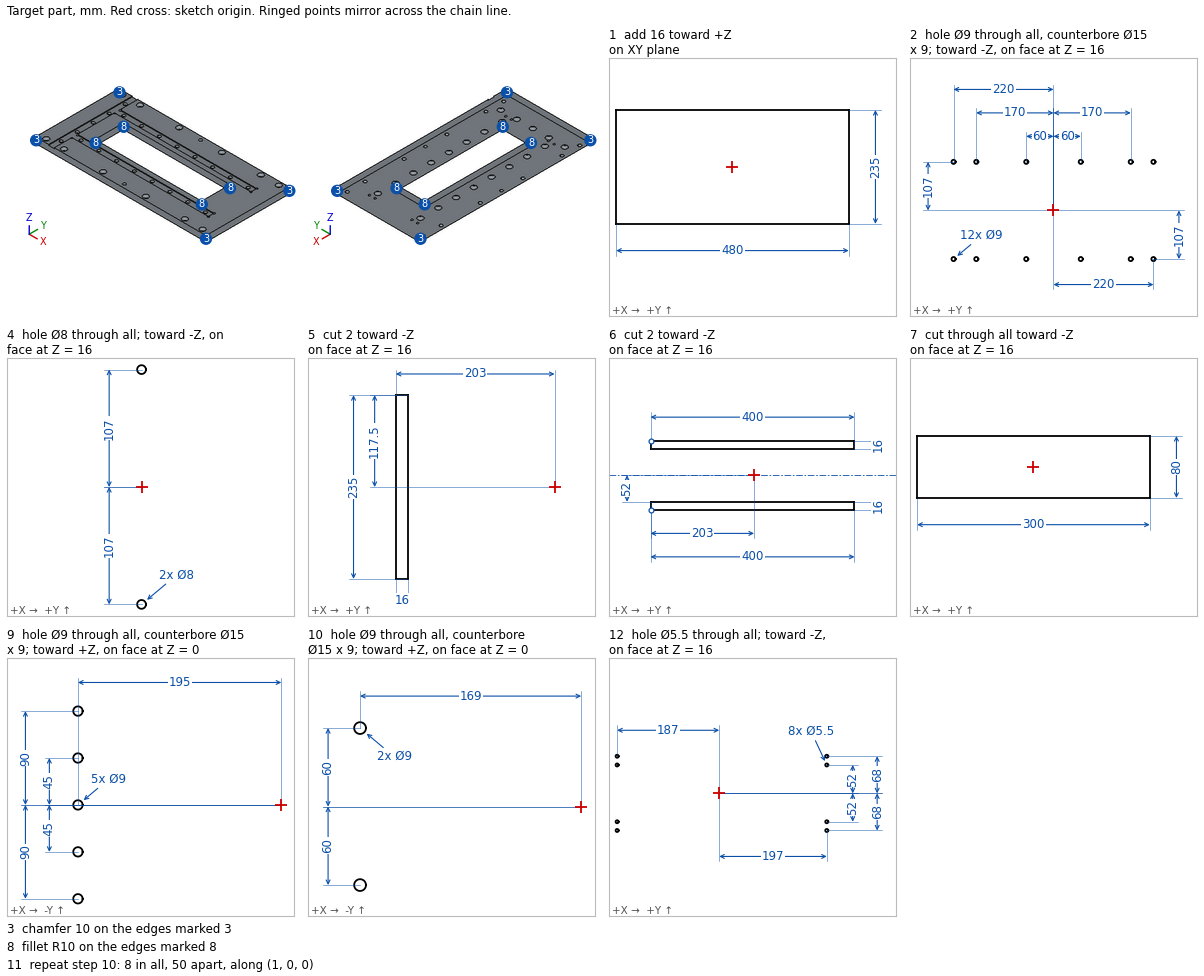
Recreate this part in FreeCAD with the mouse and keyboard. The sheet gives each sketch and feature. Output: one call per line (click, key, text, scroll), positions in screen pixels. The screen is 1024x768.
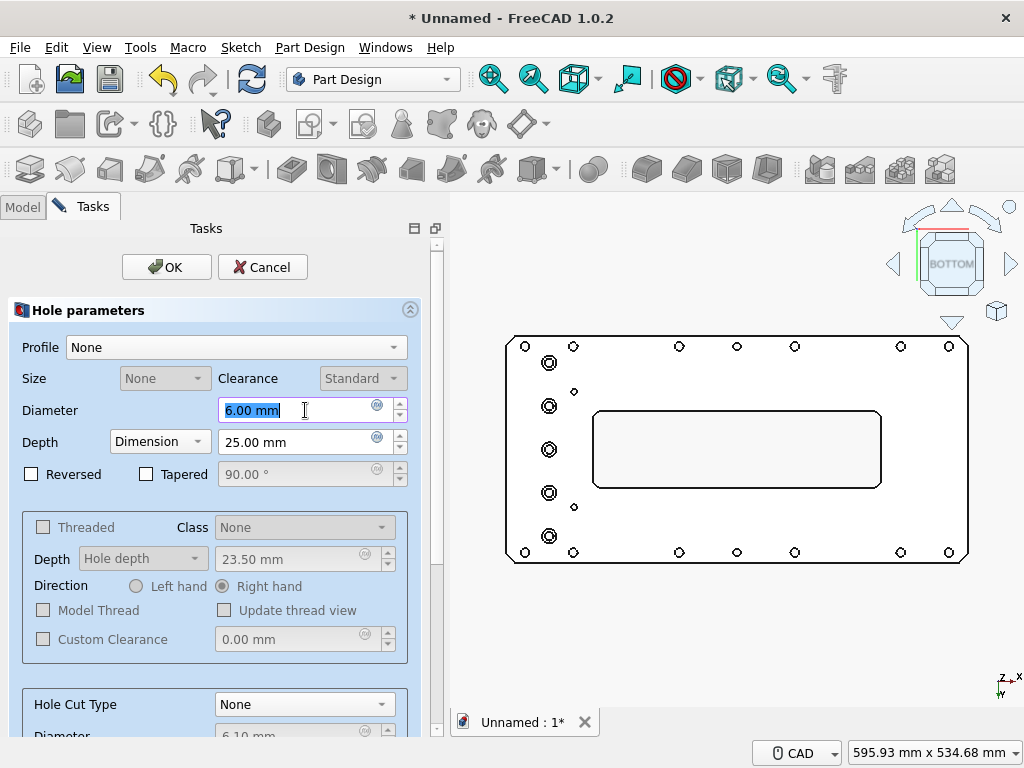
text(9)
key(Tab)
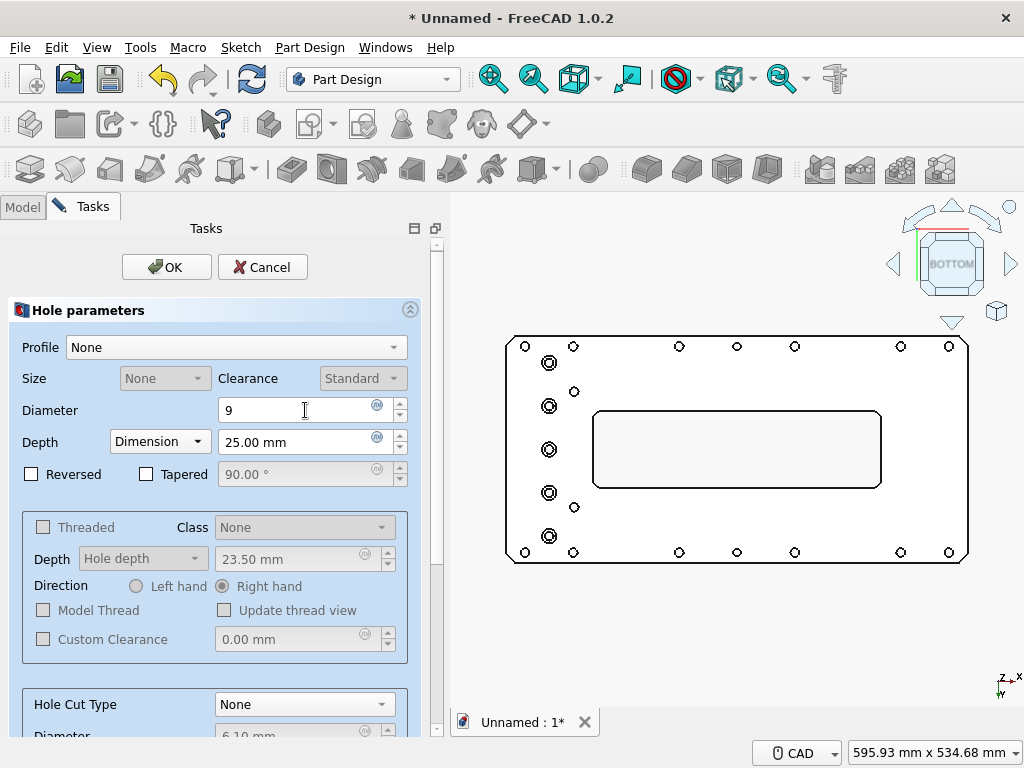
click(161, 442)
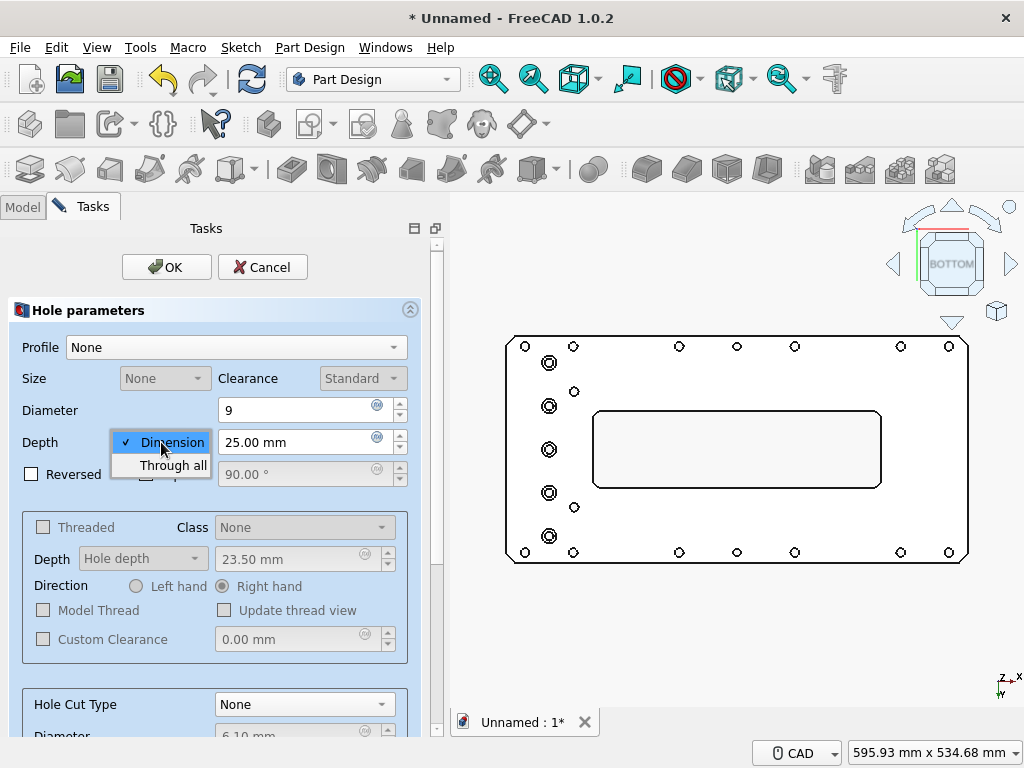
click(160, 466)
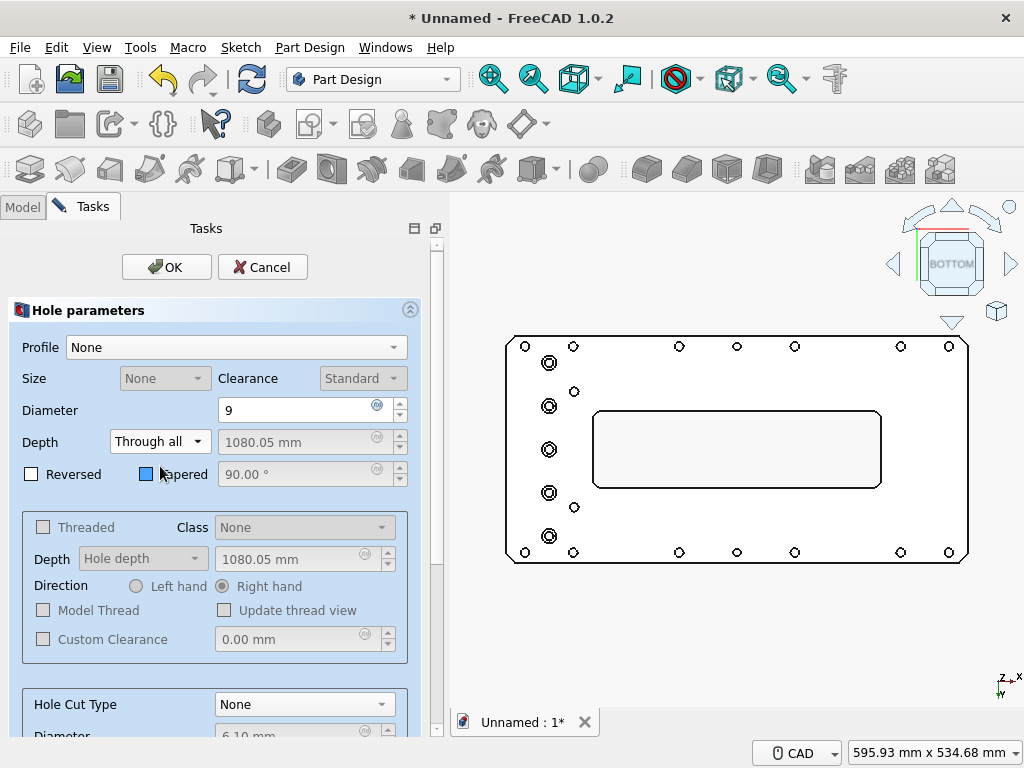
click(306, 704)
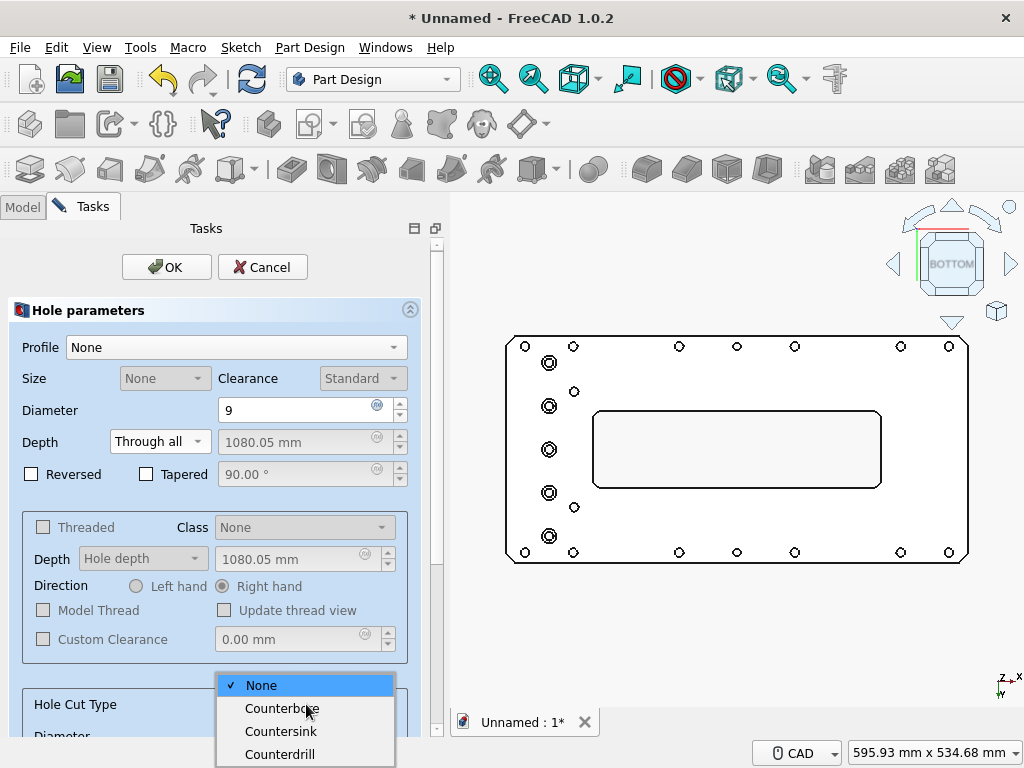
click(304, 708)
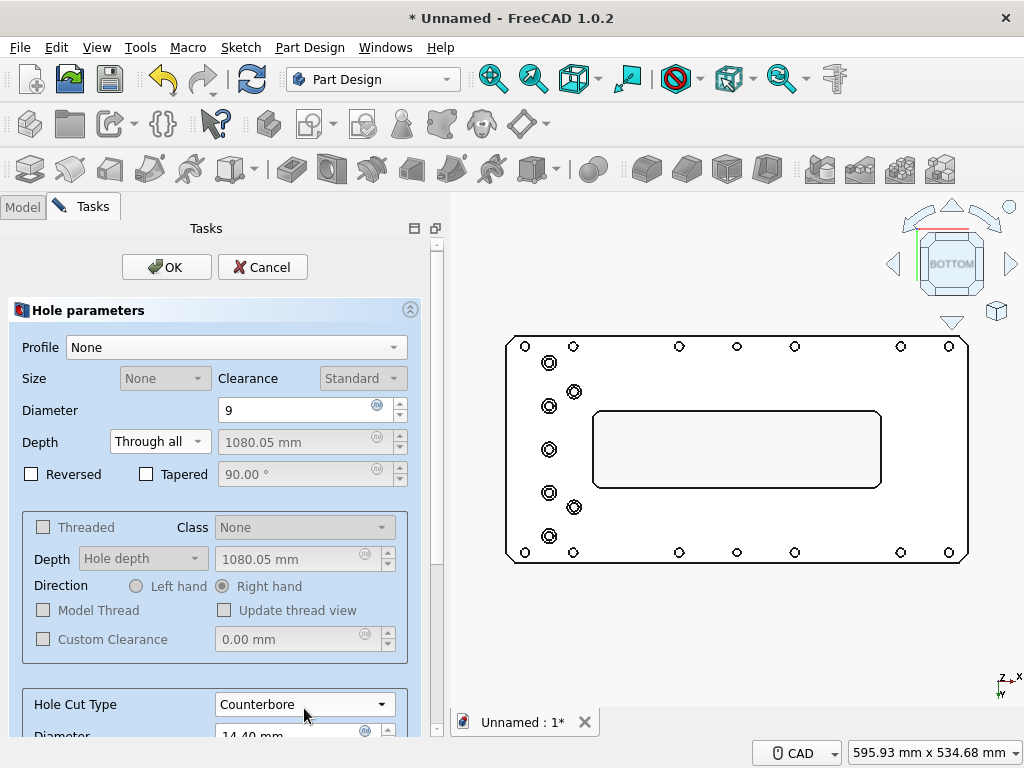
scroll(437, 487, down, 2)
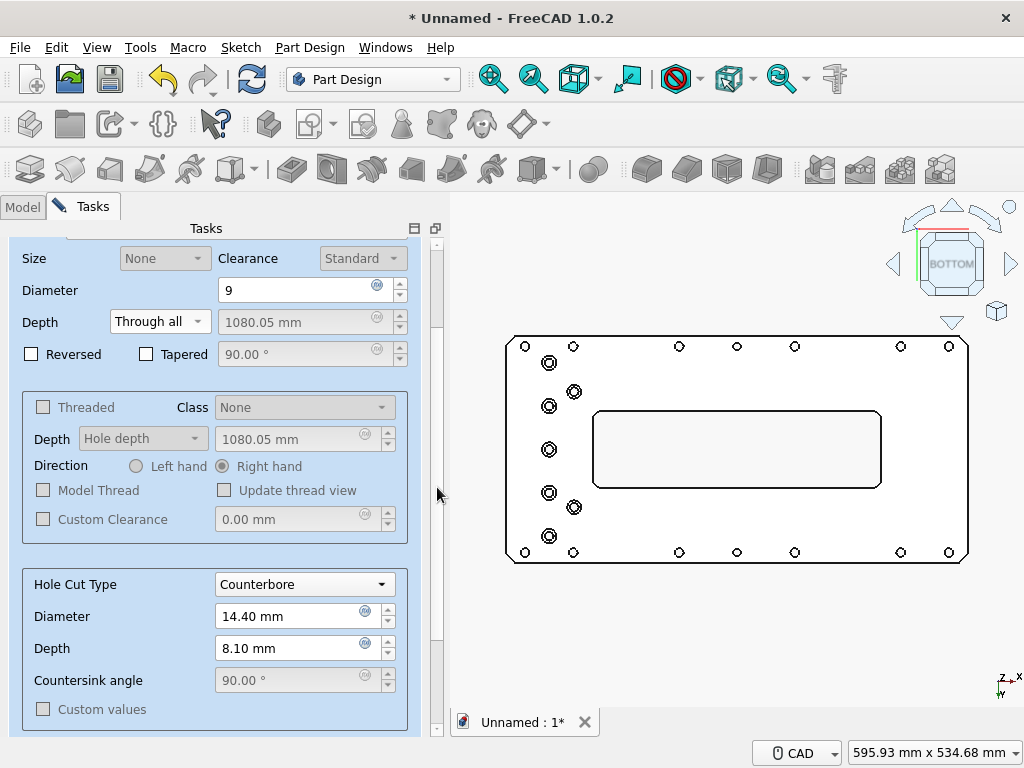
triple_click(298, 616)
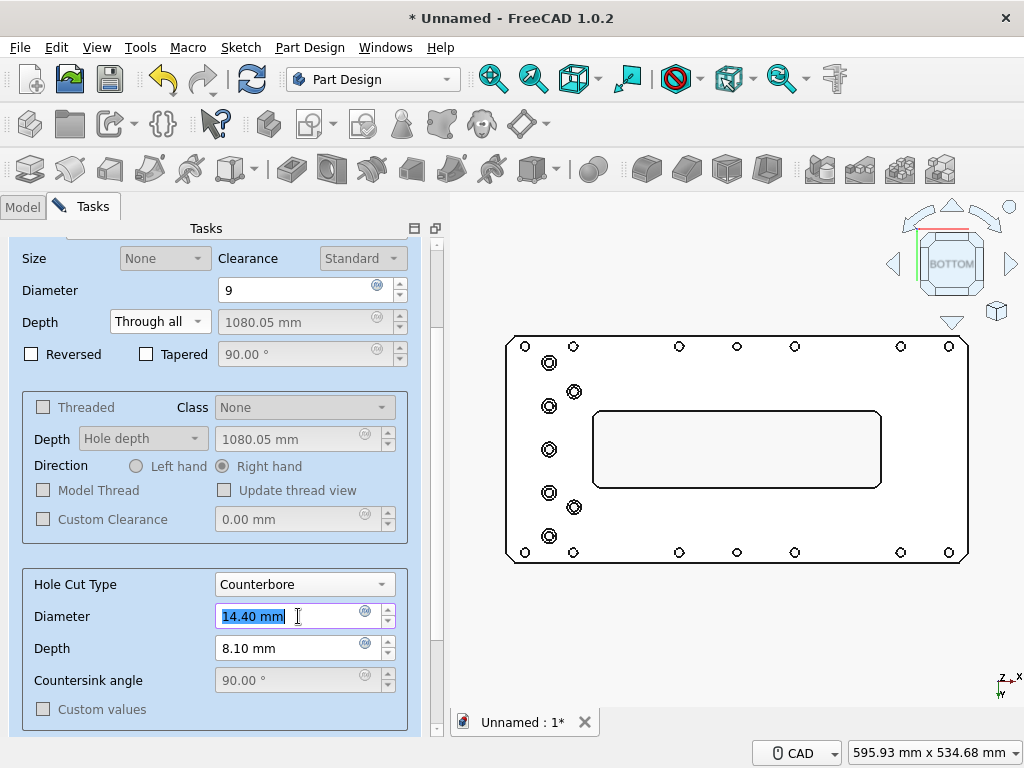
text(15)
key(Tab)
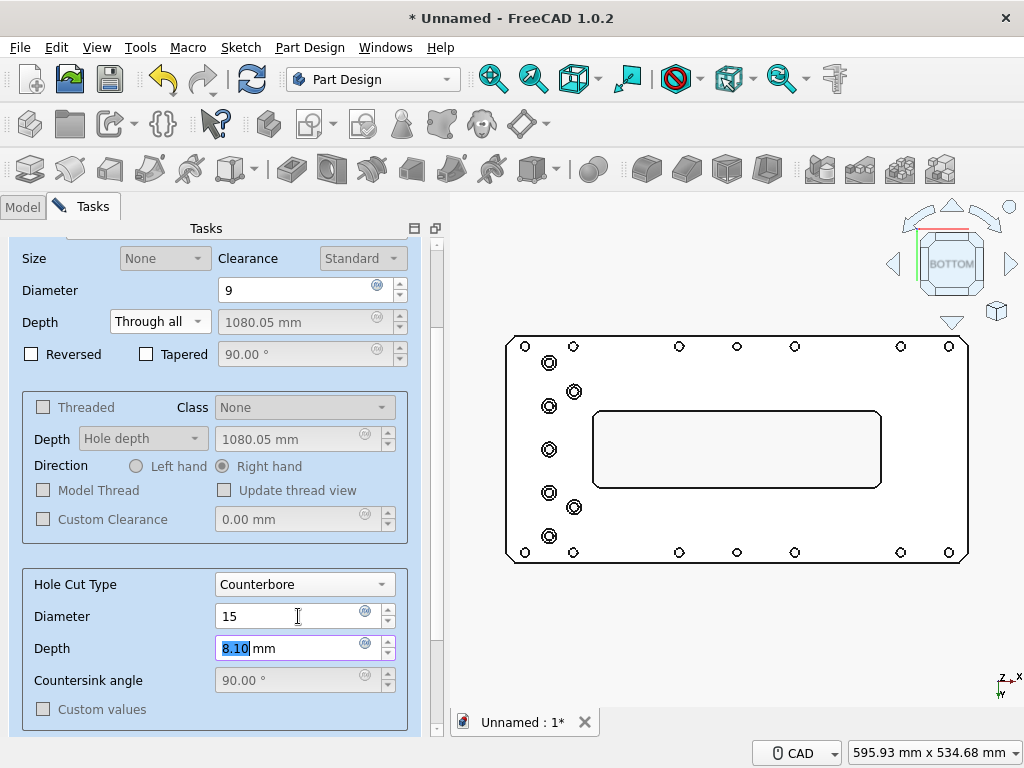
text(9)
key(Tab)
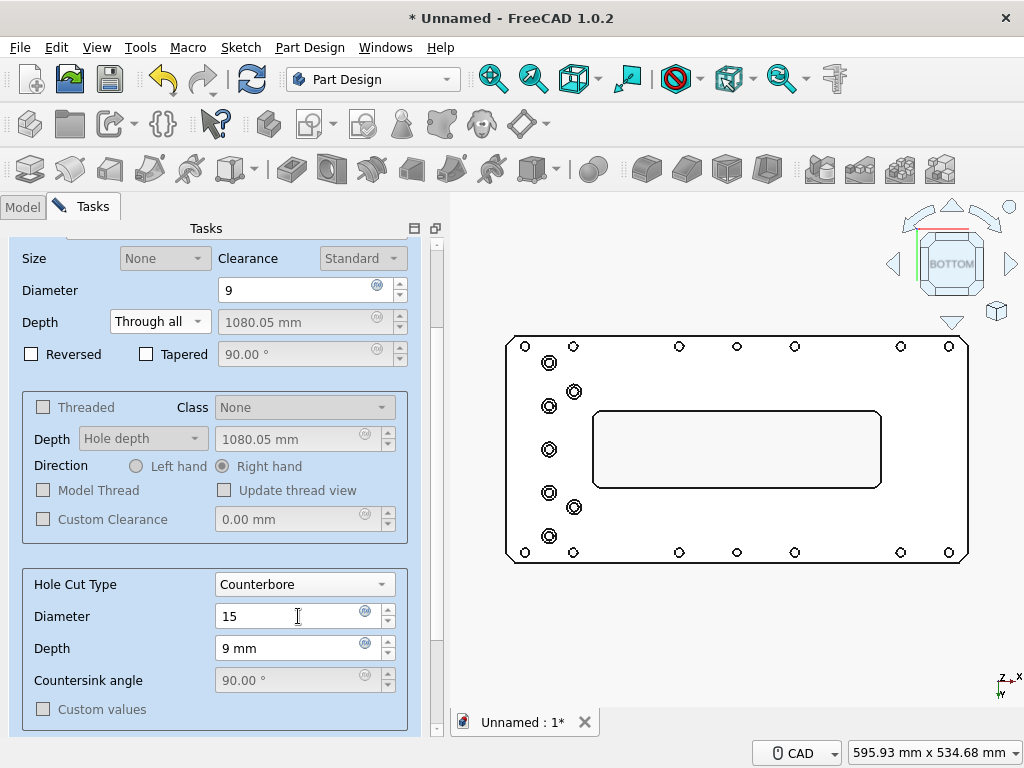
scroll(437, 487, up, 3)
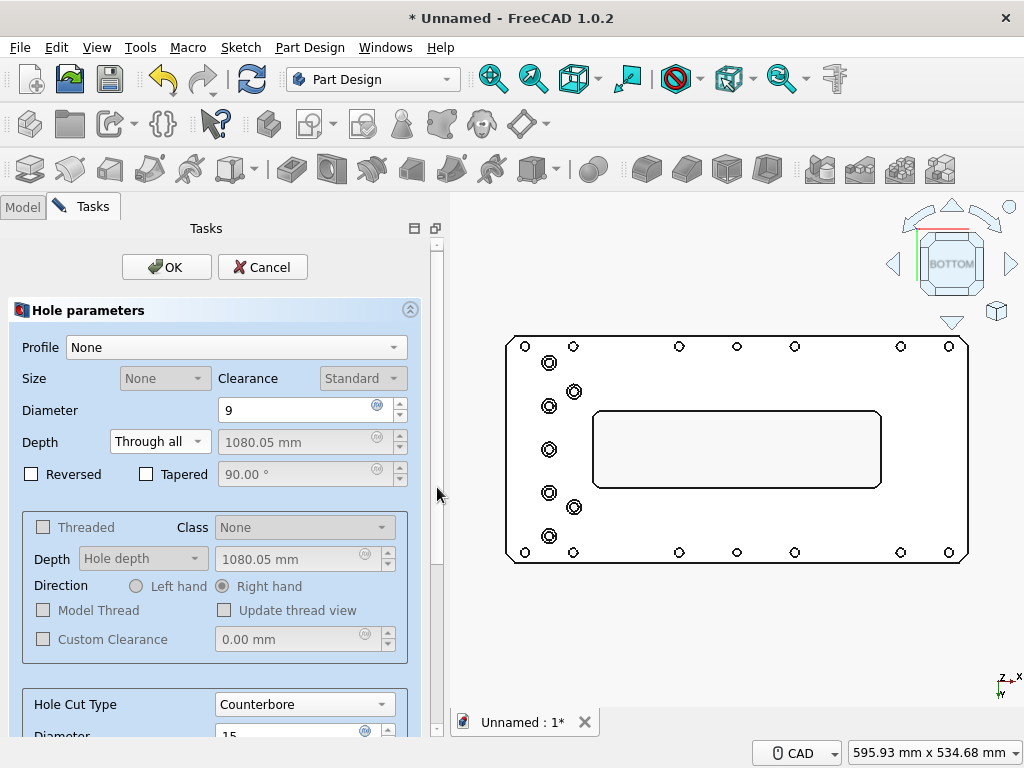
click(167, 267)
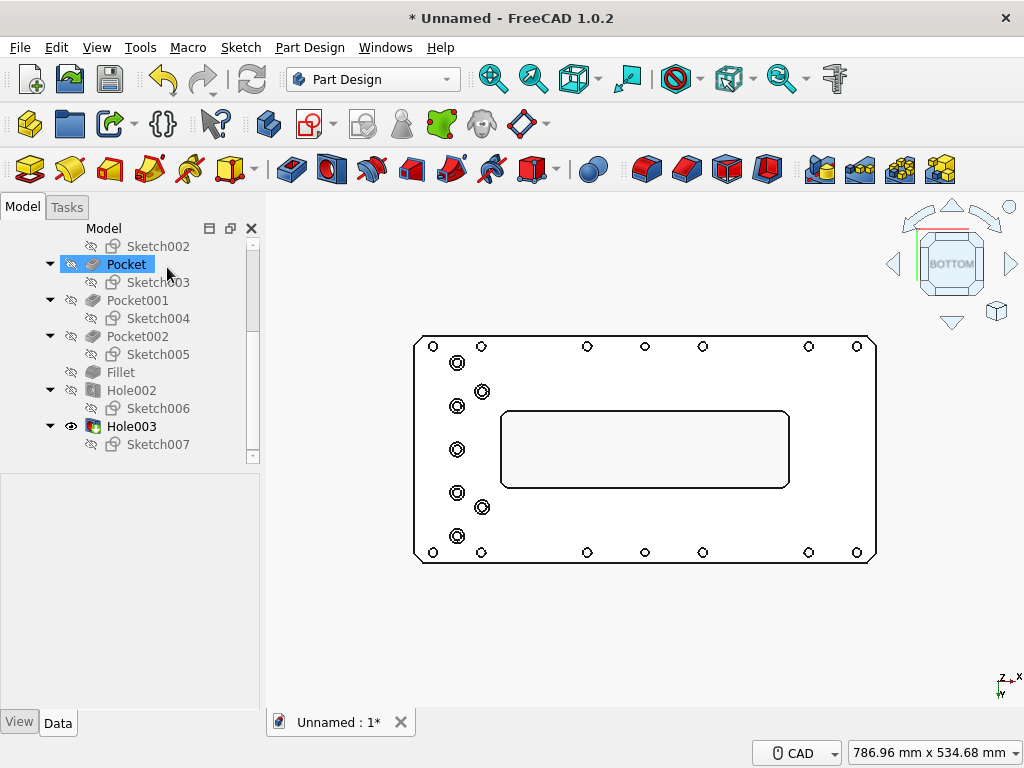
click(116, 426)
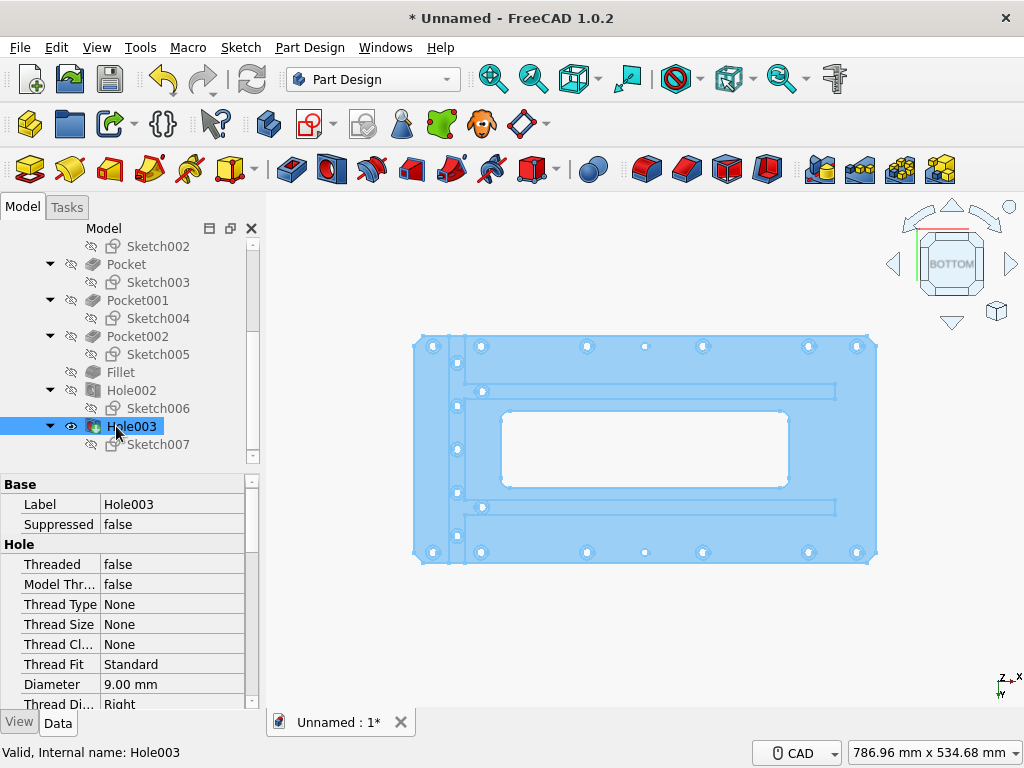
click(860, 170)